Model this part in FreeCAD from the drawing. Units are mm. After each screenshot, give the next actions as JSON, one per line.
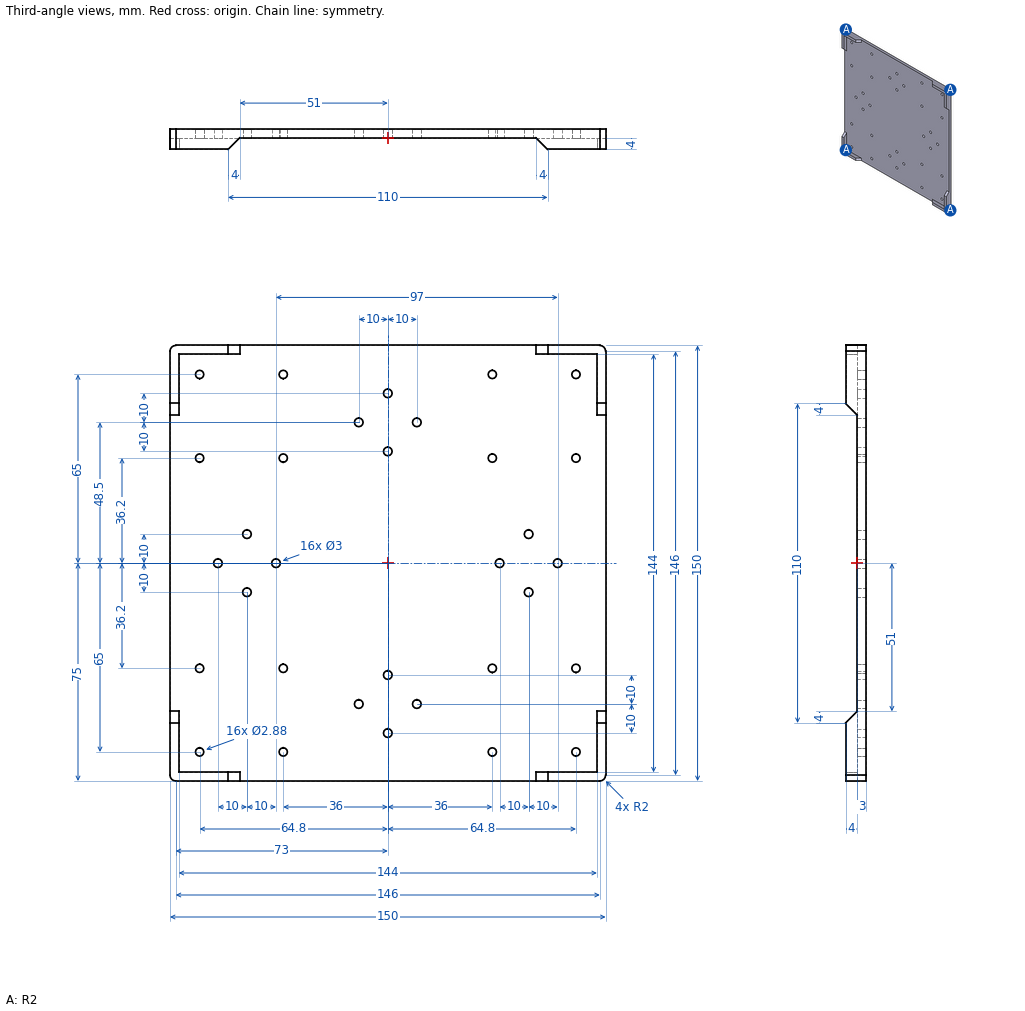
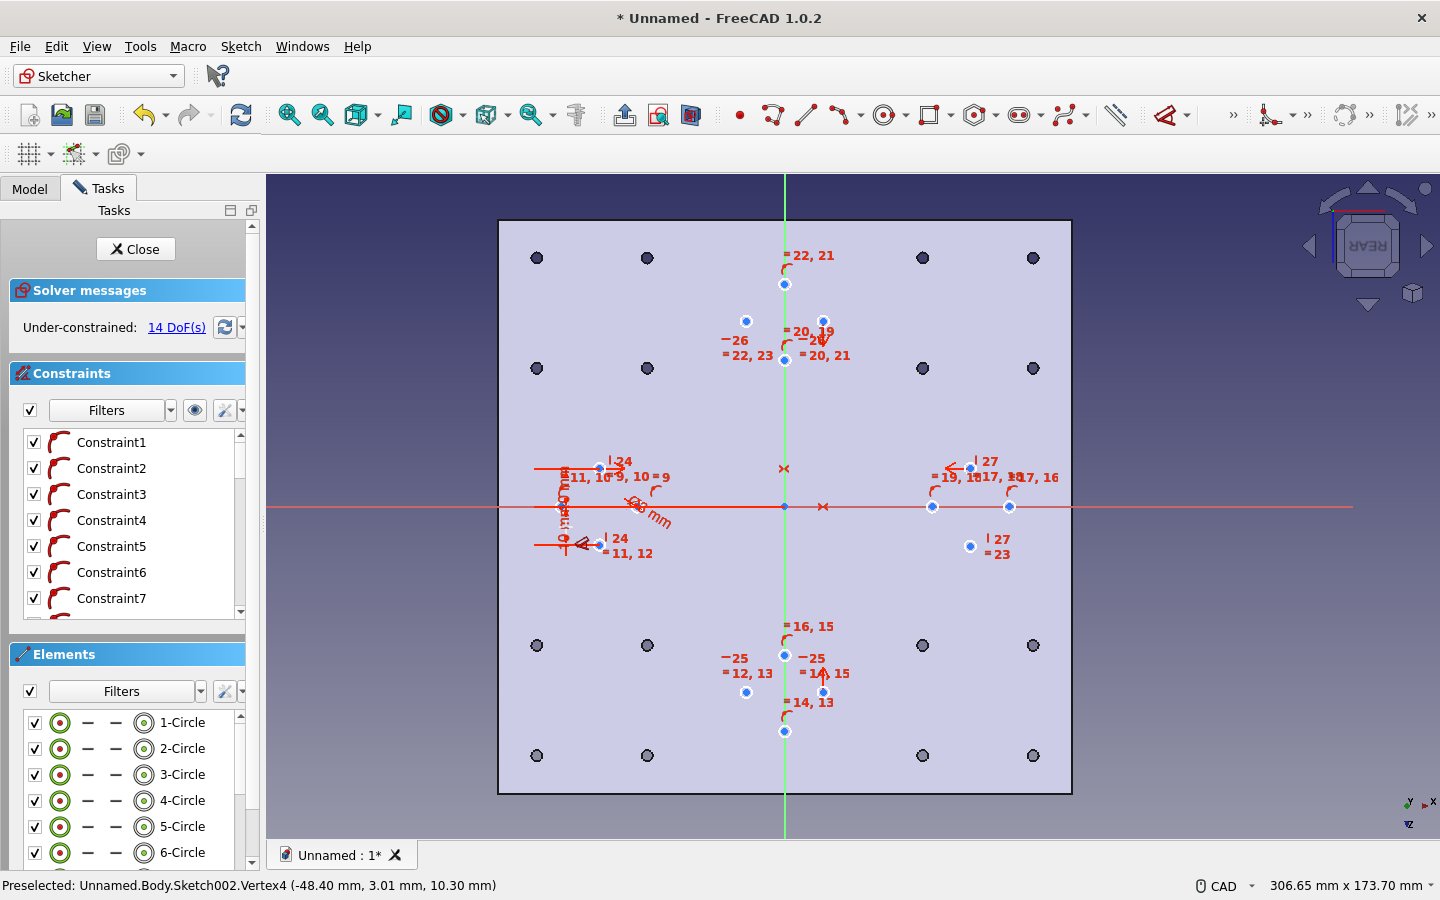
{"action": "left_click", "coordinate": [746, 692]}
{"action": "left_click", "coordinate": [766, 726]}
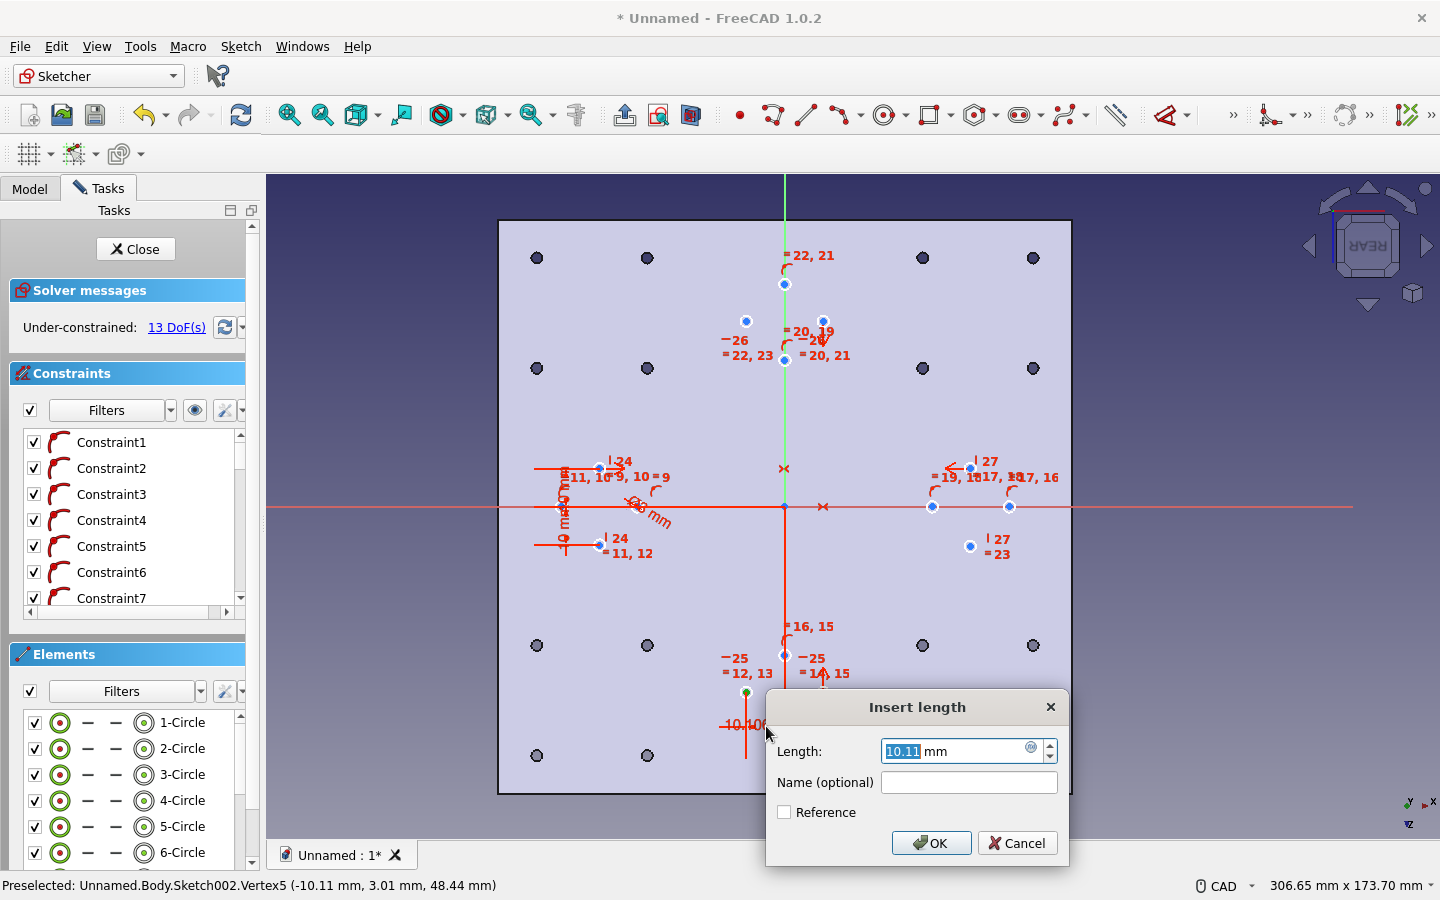
{"action": "type", "text": "10"}
{"action": "key", "text": "Return"}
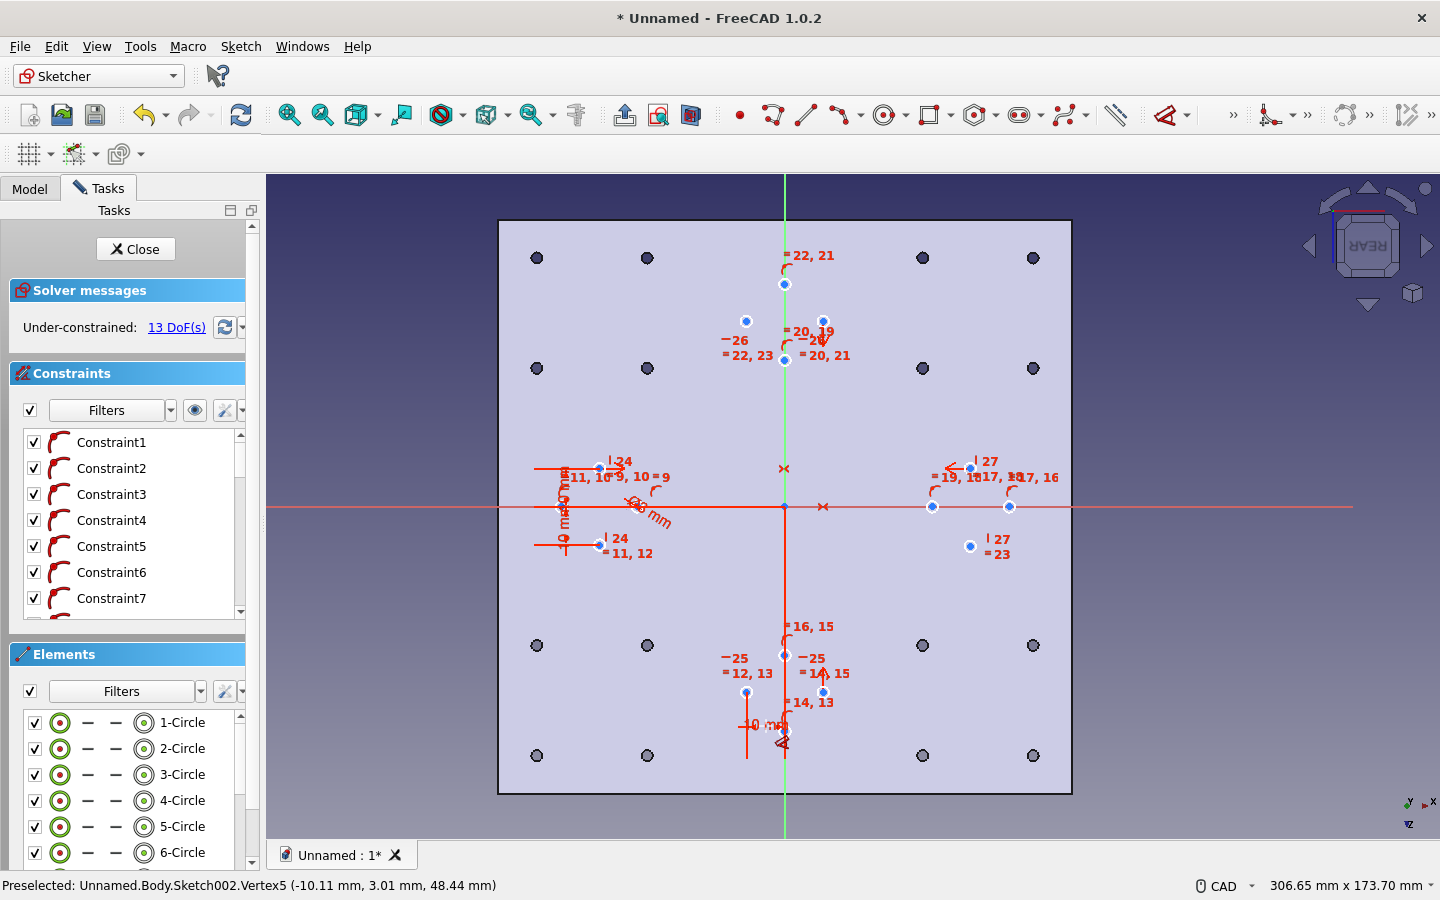
{"action": "left_click", "coordinate": [823, 692]}
{"action": "left_click", "coordinate": [804, 473]}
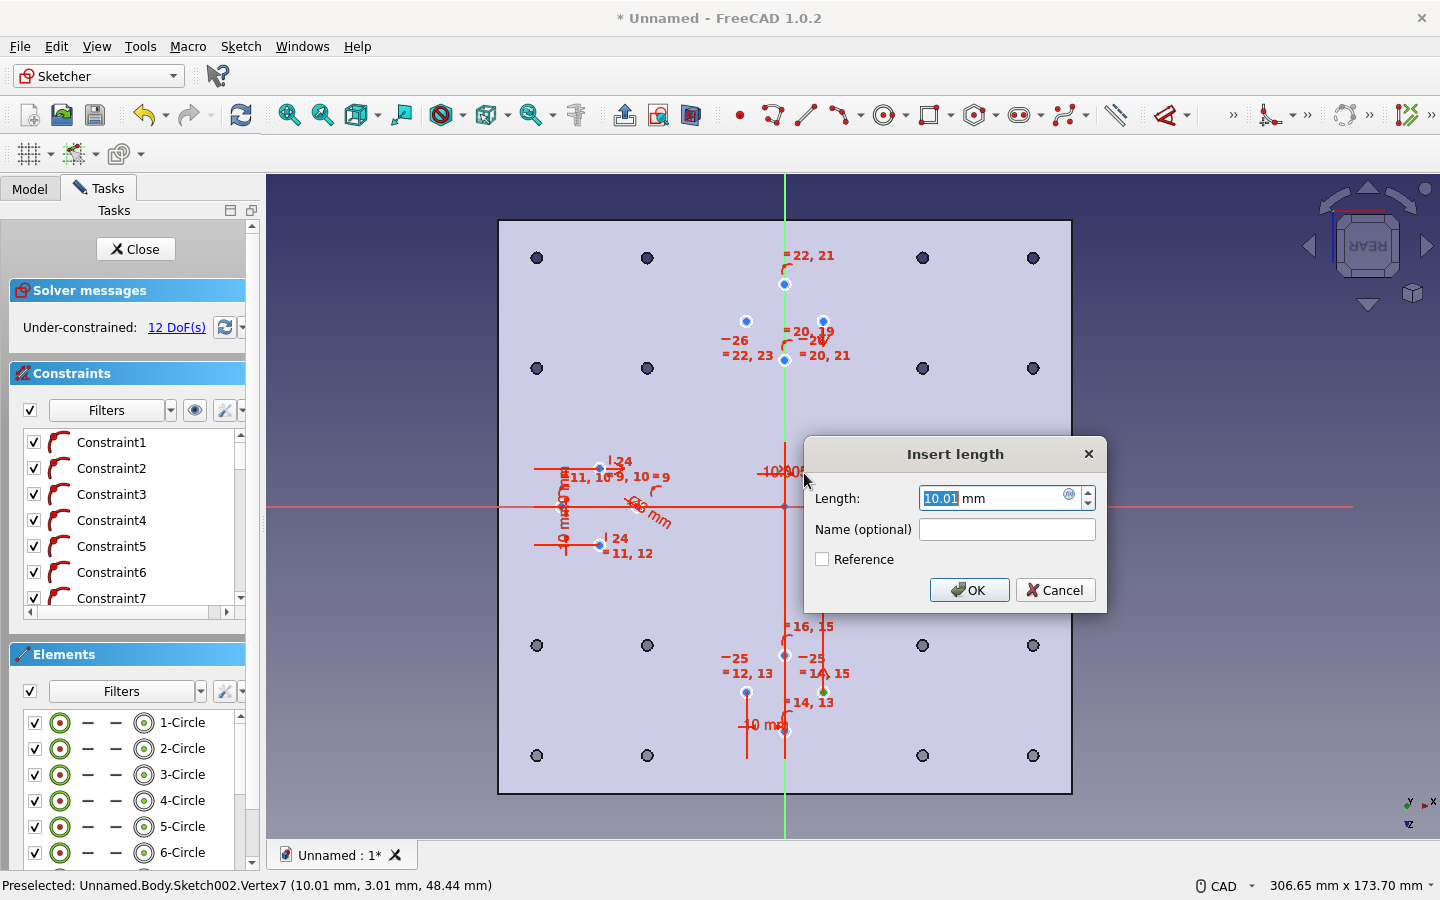
{"action": "type", "text": "10"}
{"action": "key", "text": "Return"}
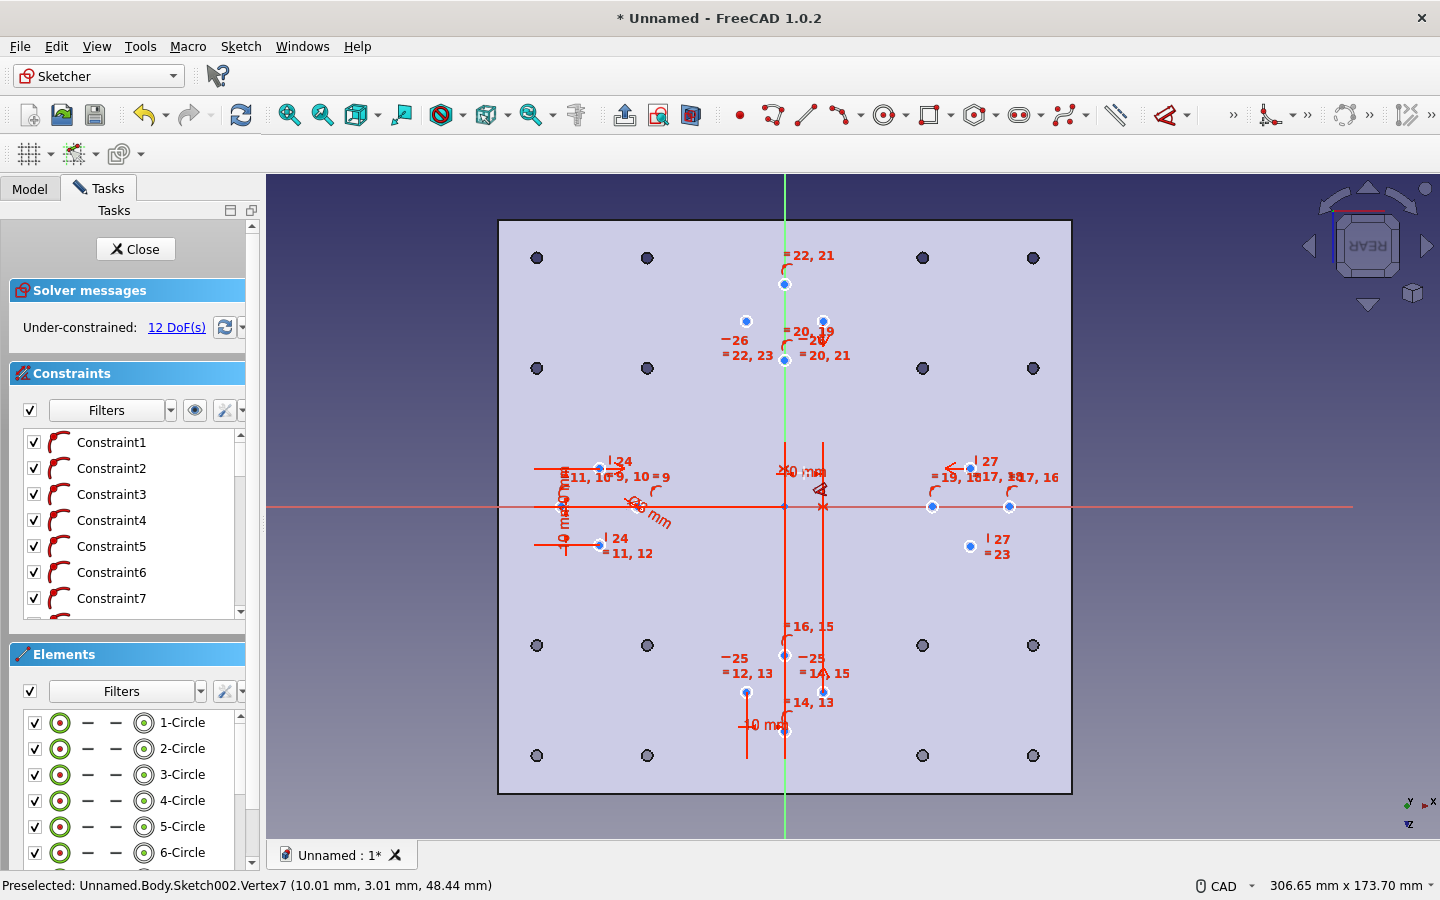
{"action": "left_click", "coordinate": [746, 321]}
{"action": "left_click", "coordinate": [766, 287]}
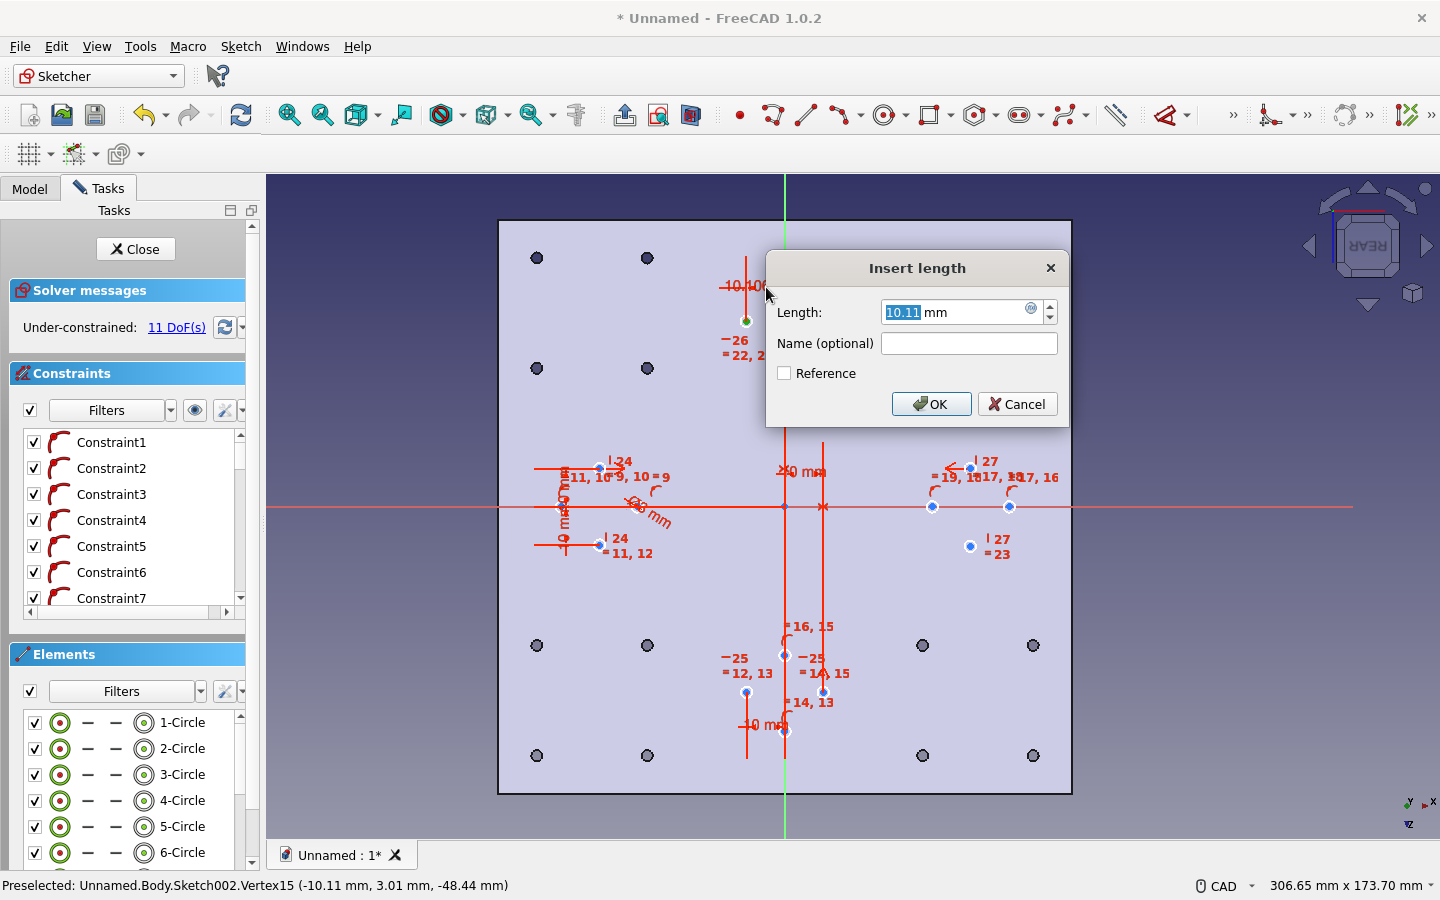
{"action": "type", "text": "10"}
{"action": "key", "text": "Return"}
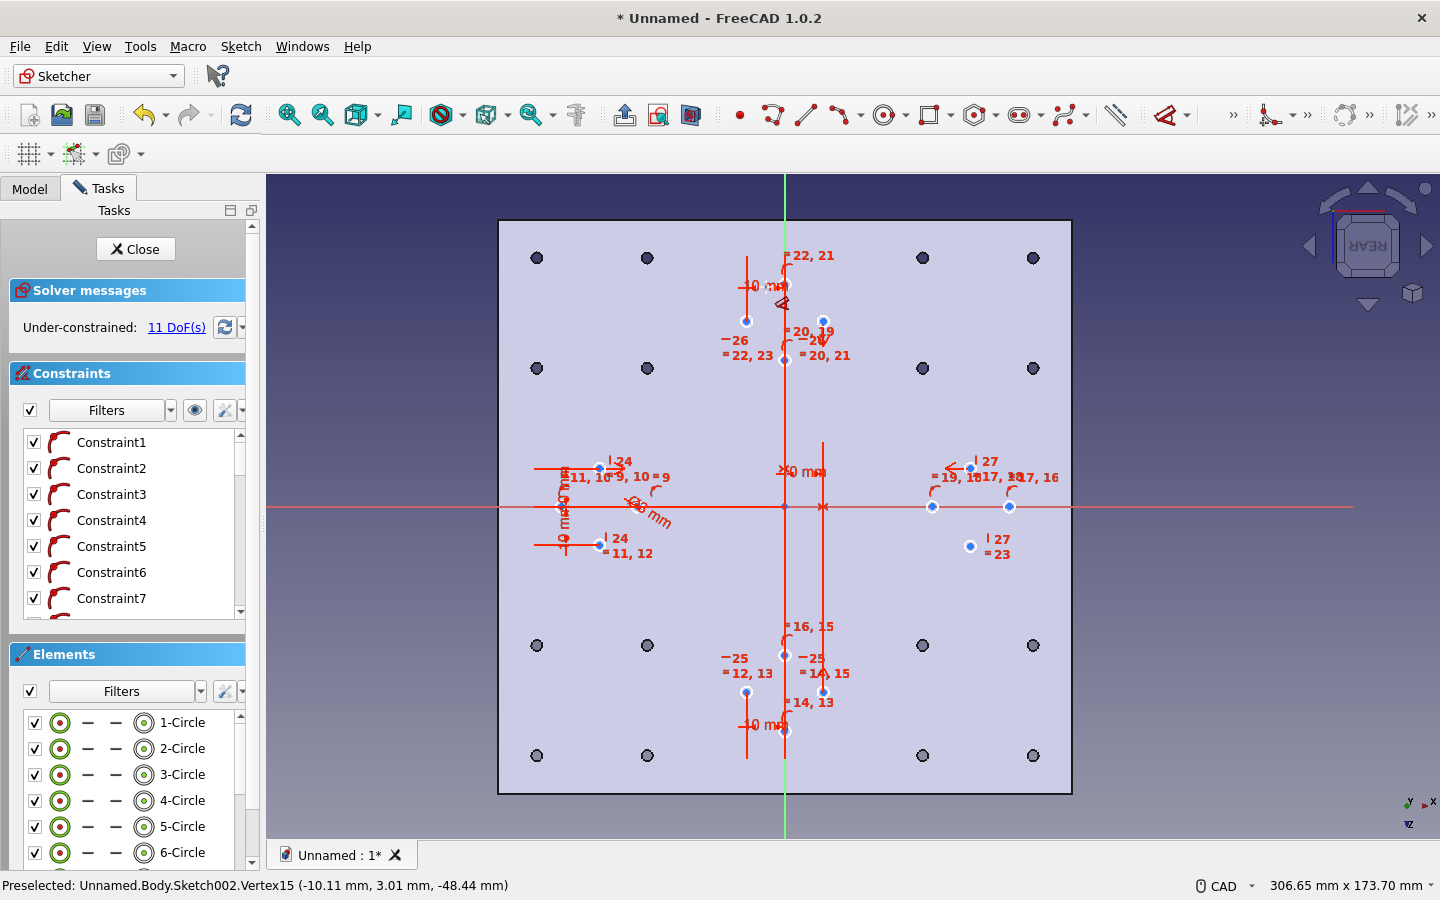
{"action": "left_click", "coordinate": [970, 546]}
{"action": "left_click", "coordinate": [1004, 527]}